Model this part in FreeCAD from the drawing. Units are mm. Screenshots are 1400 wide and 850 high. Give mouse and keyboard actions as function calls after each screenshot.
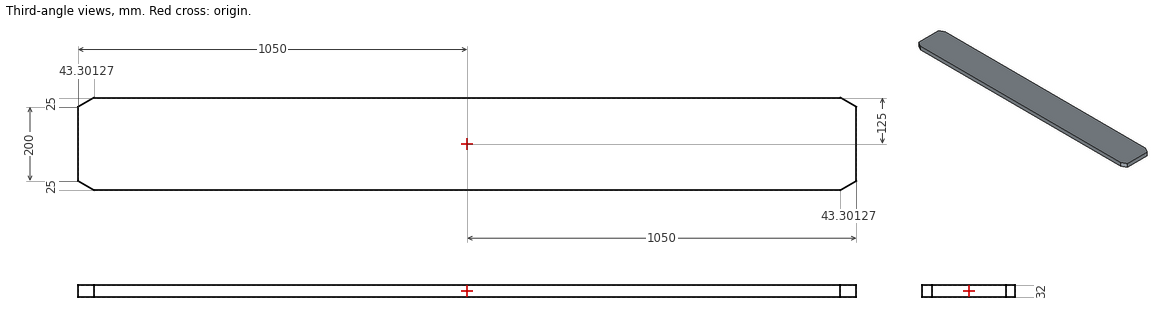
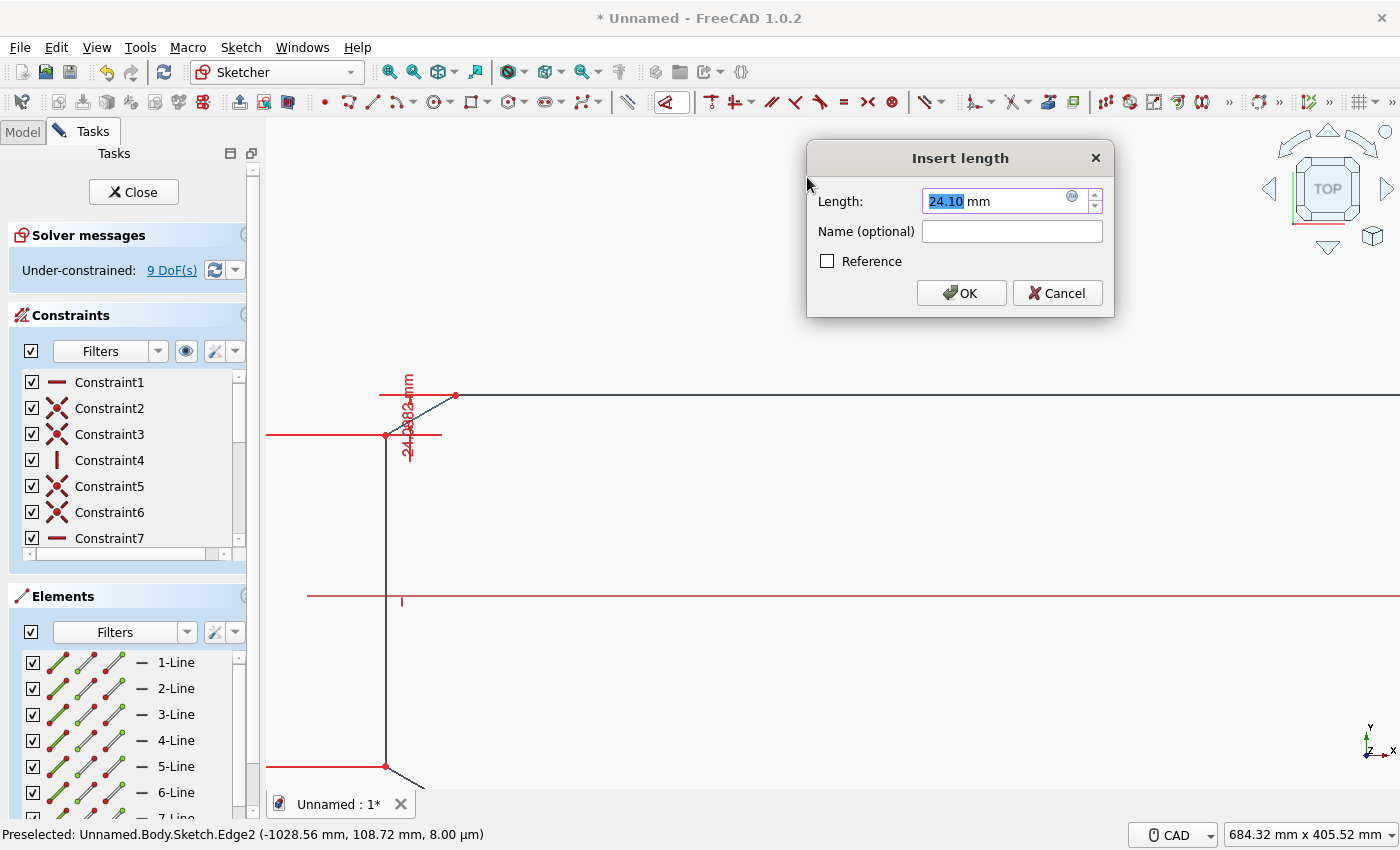
text(25)
key(Return)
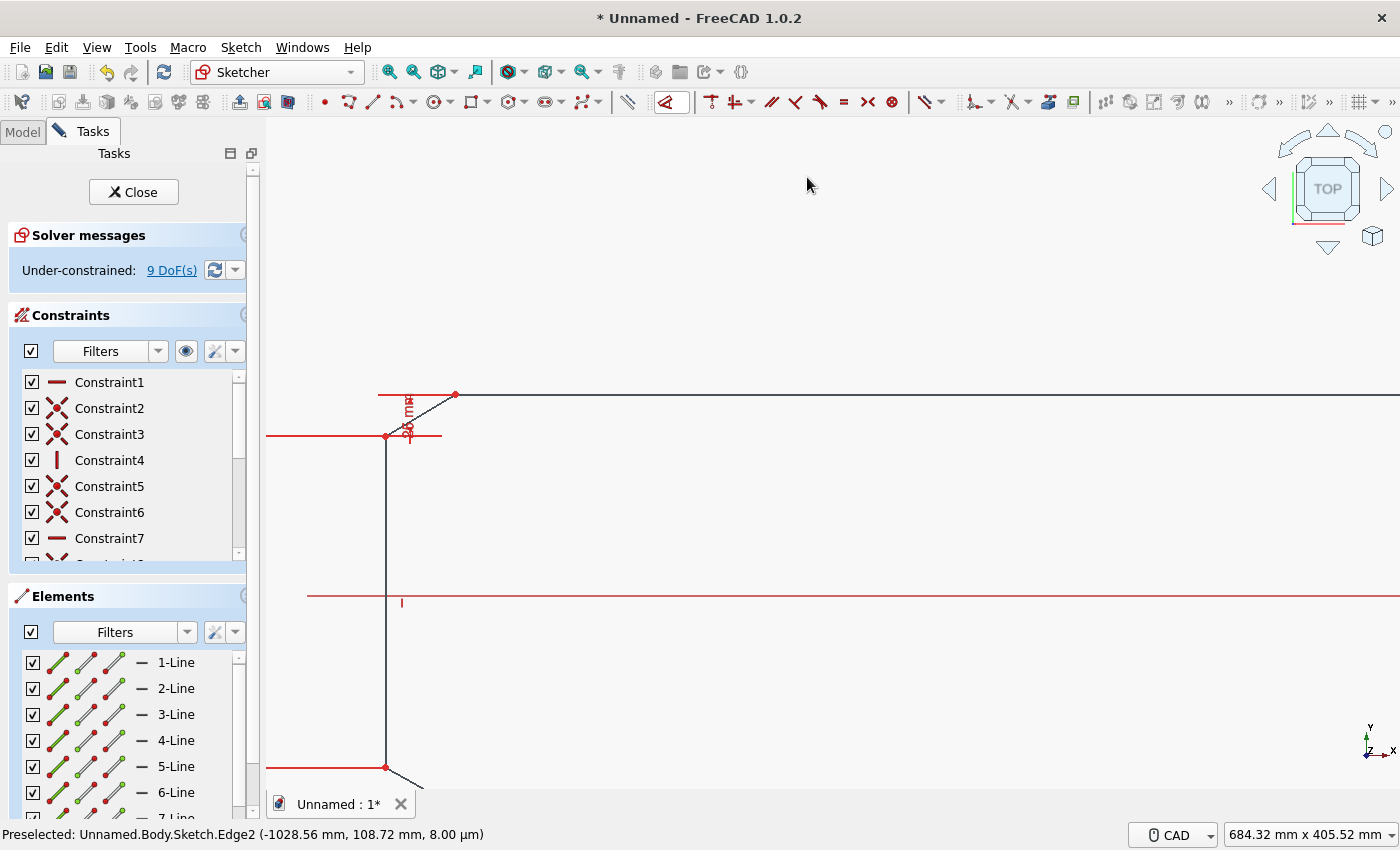
scroll(421, 417, down, 8)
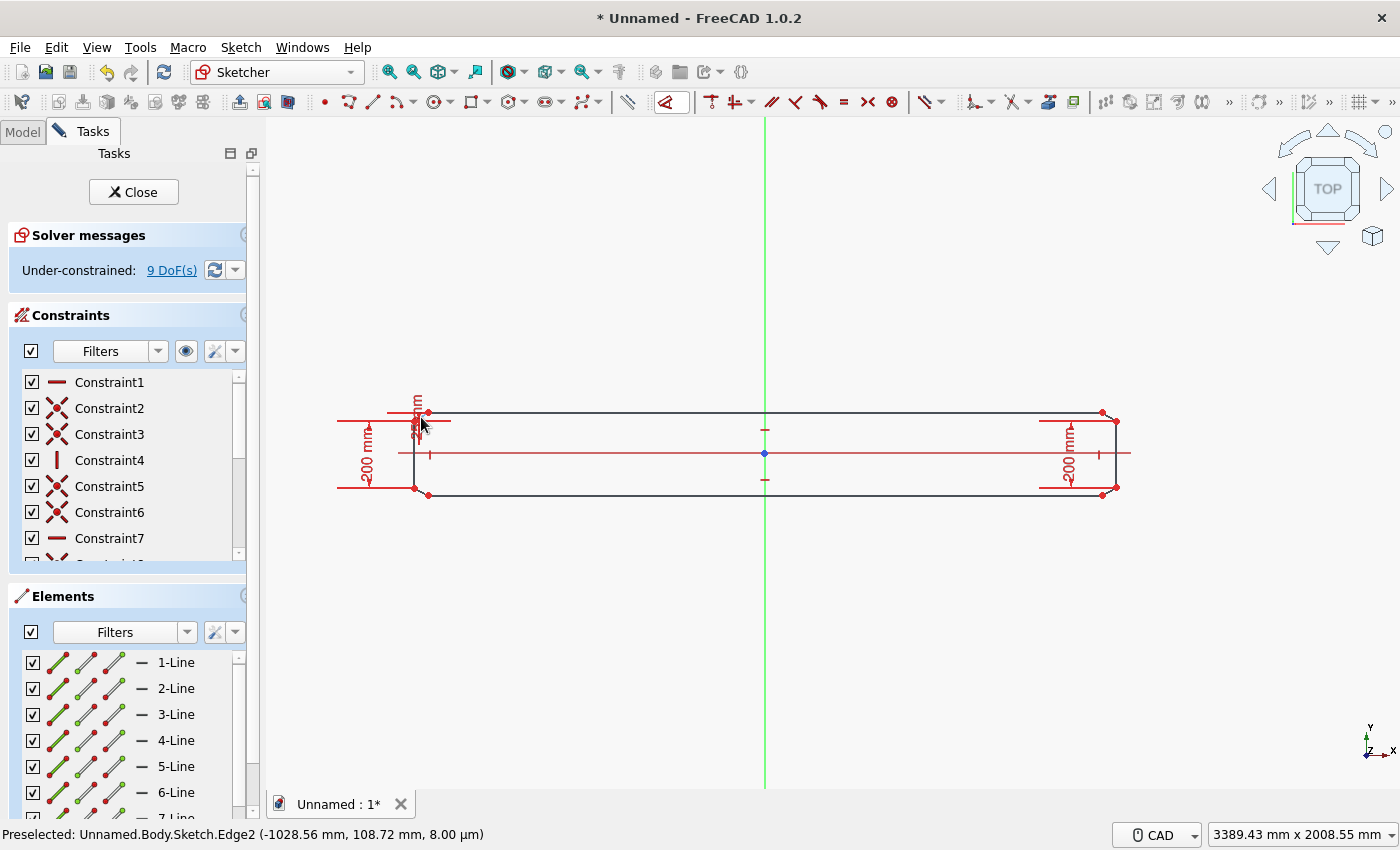
scroll(418, 491, up, 8)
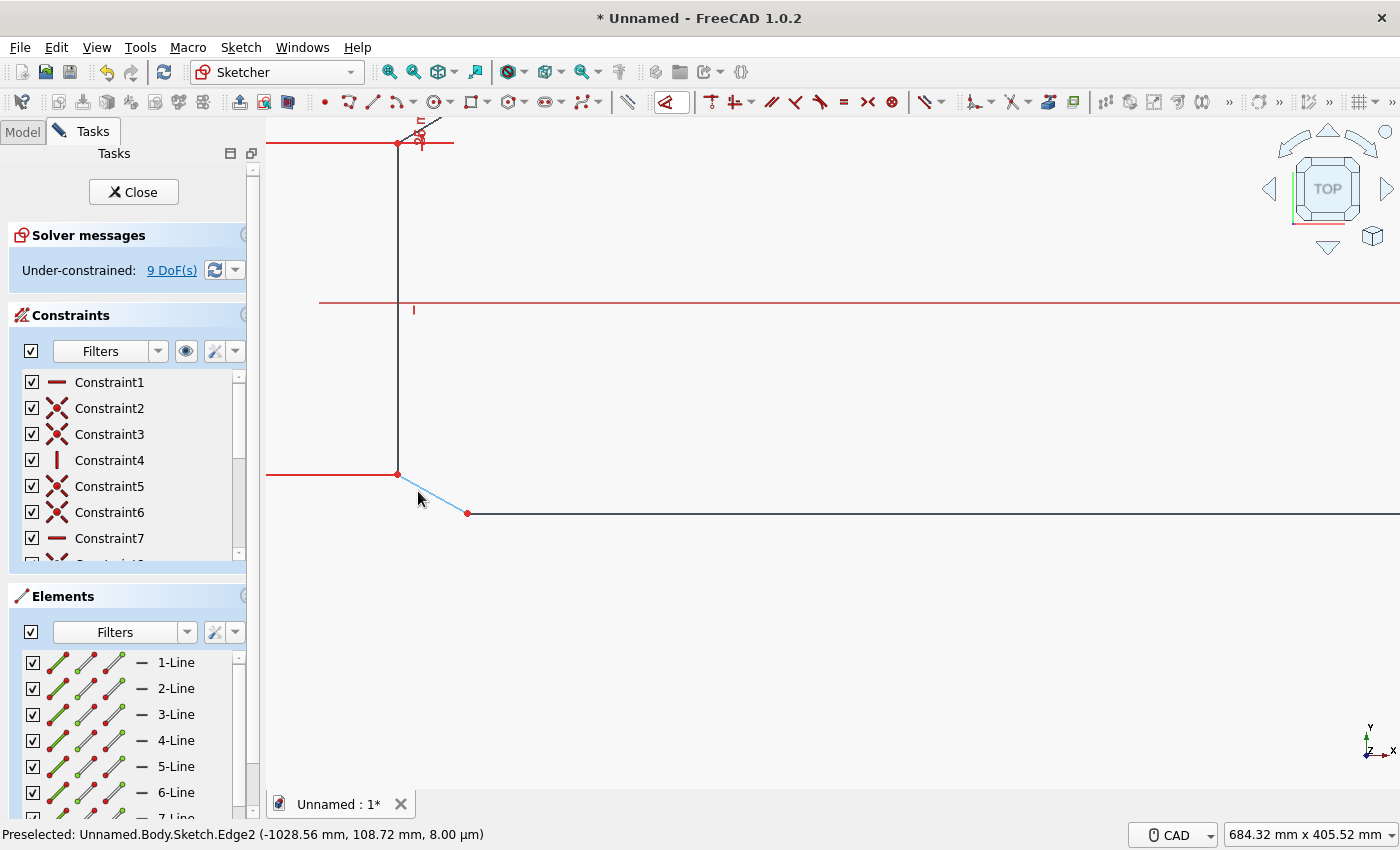
click(418, 486)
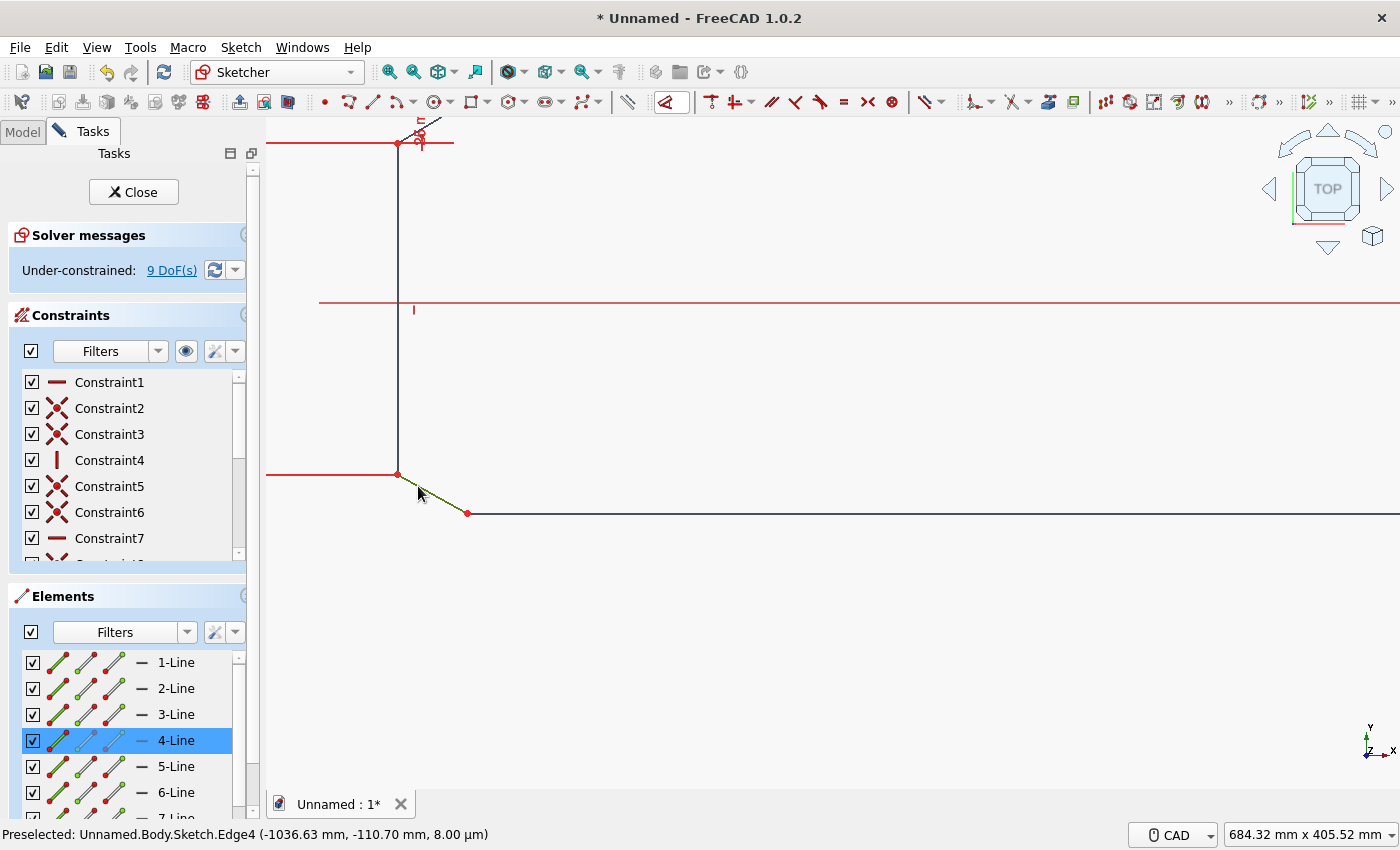
key(i)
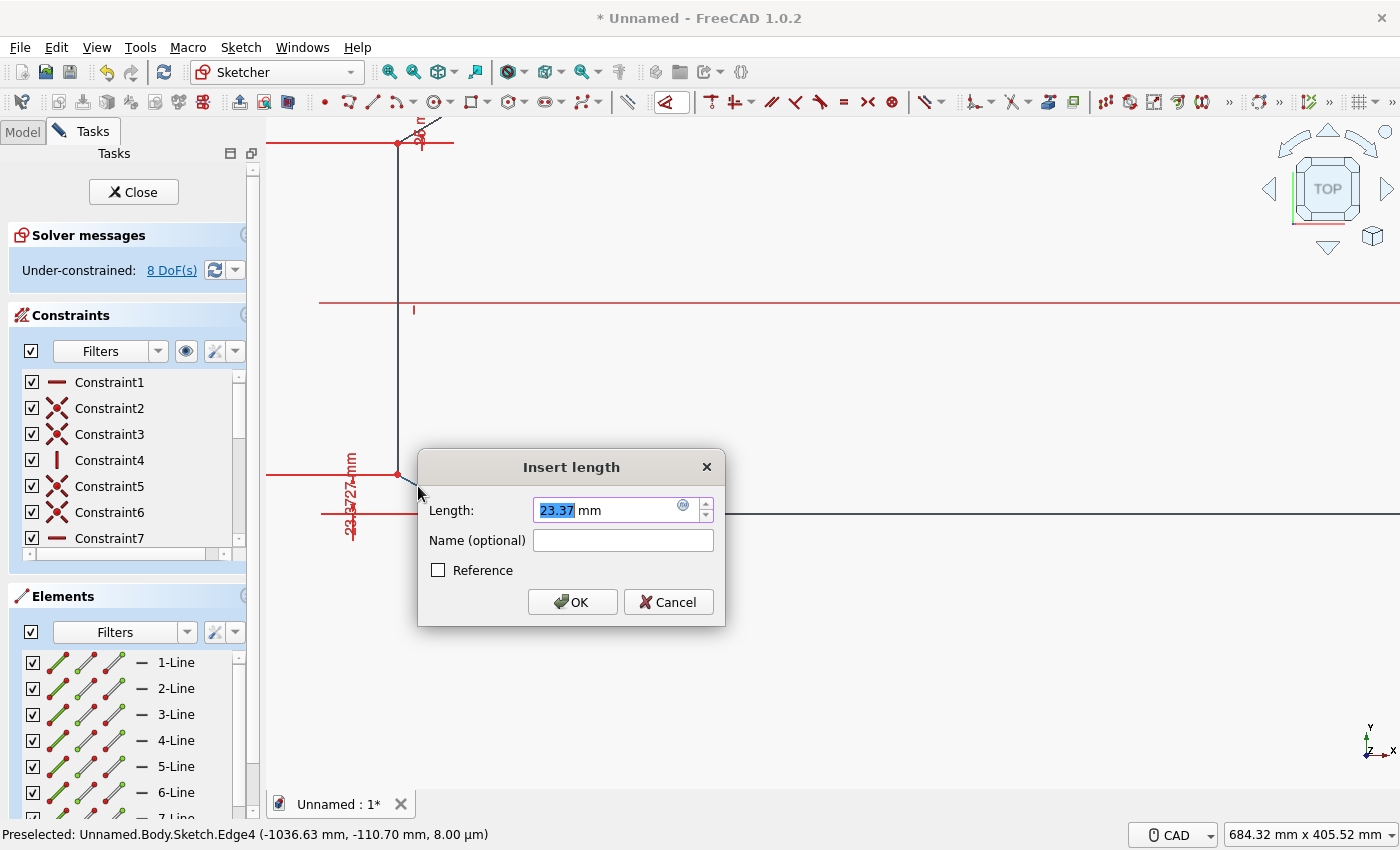
text(25)
key(Return)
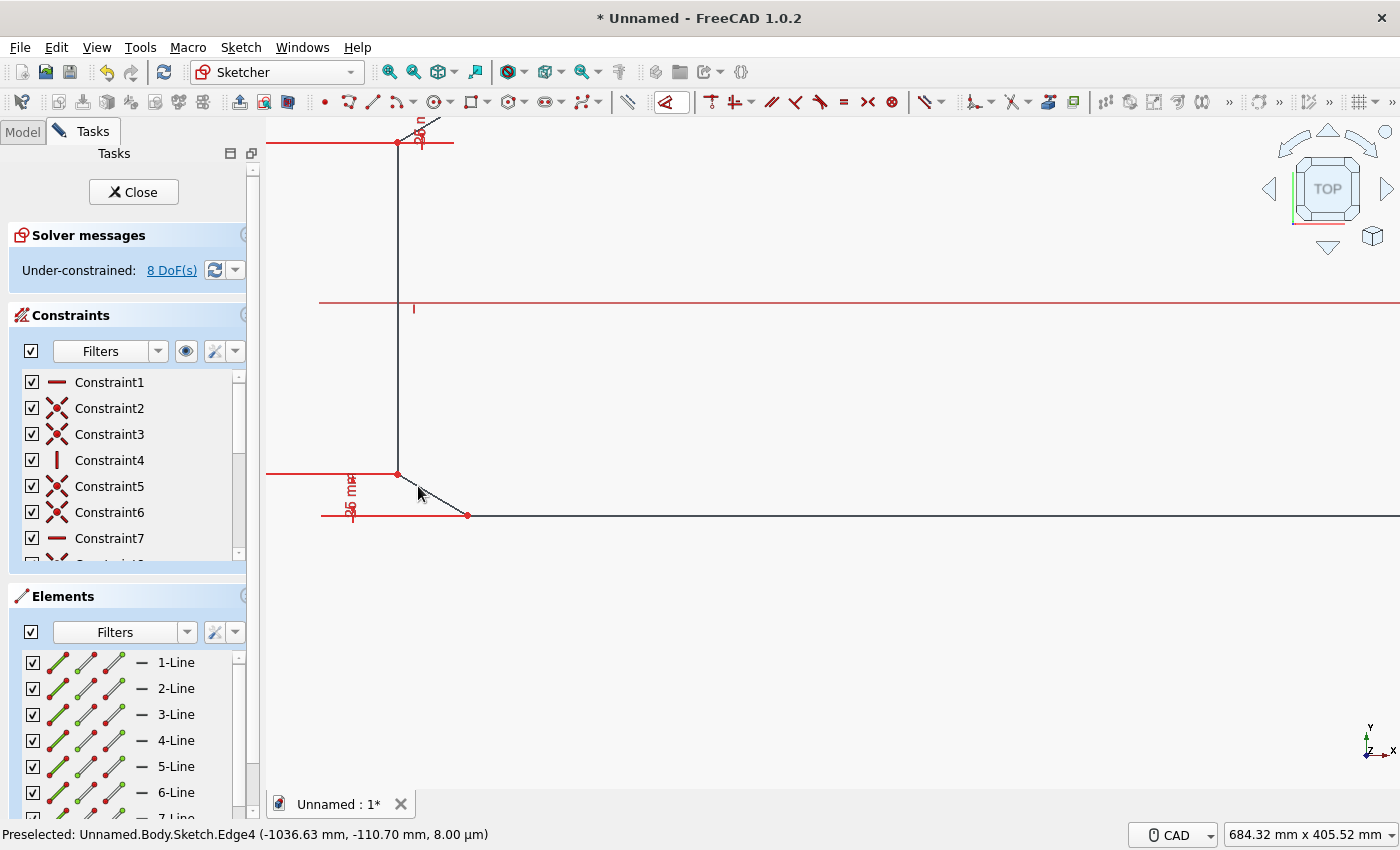
scroll(418, 491, down, 8)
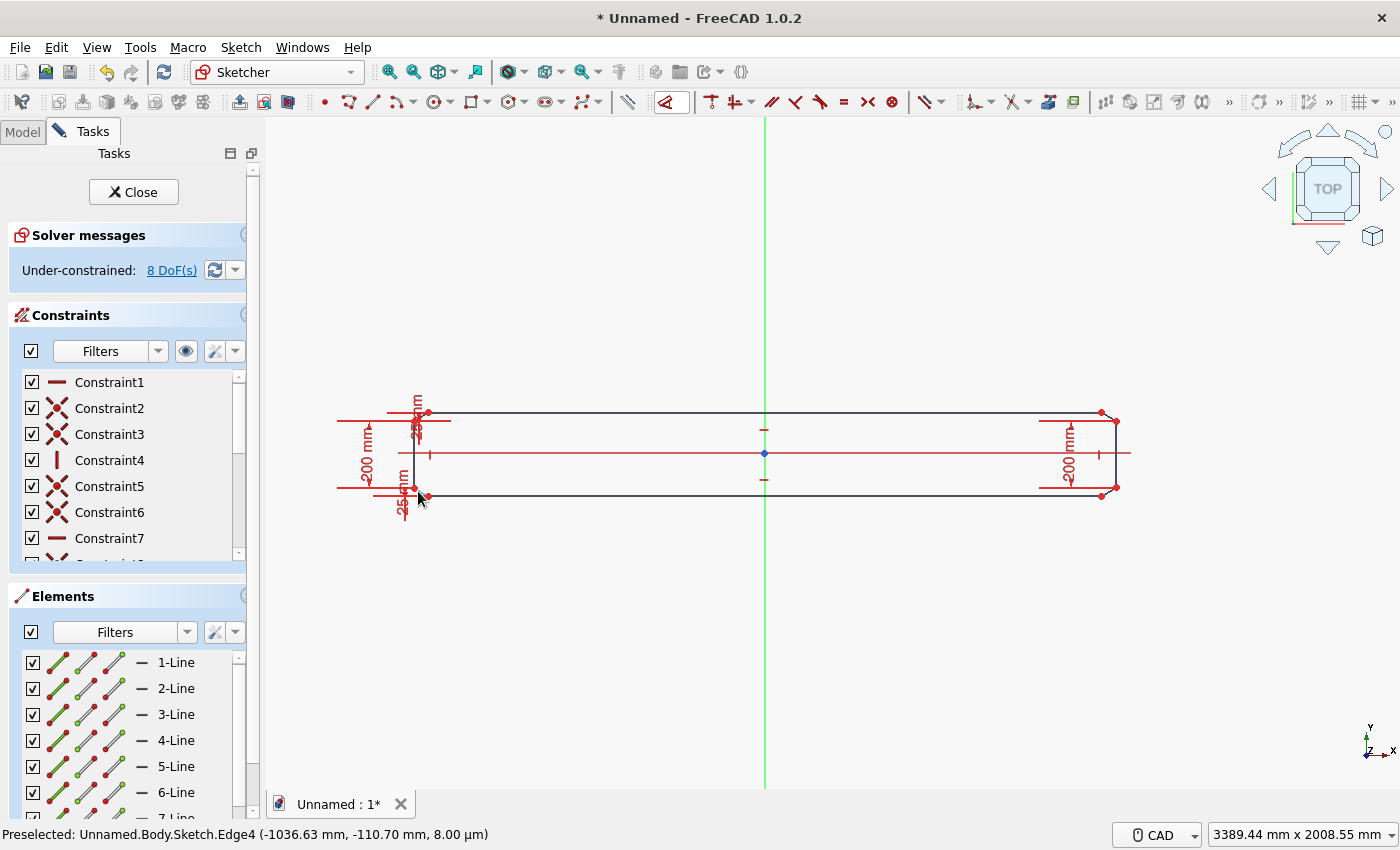
scroll(1106, 494, up, 8)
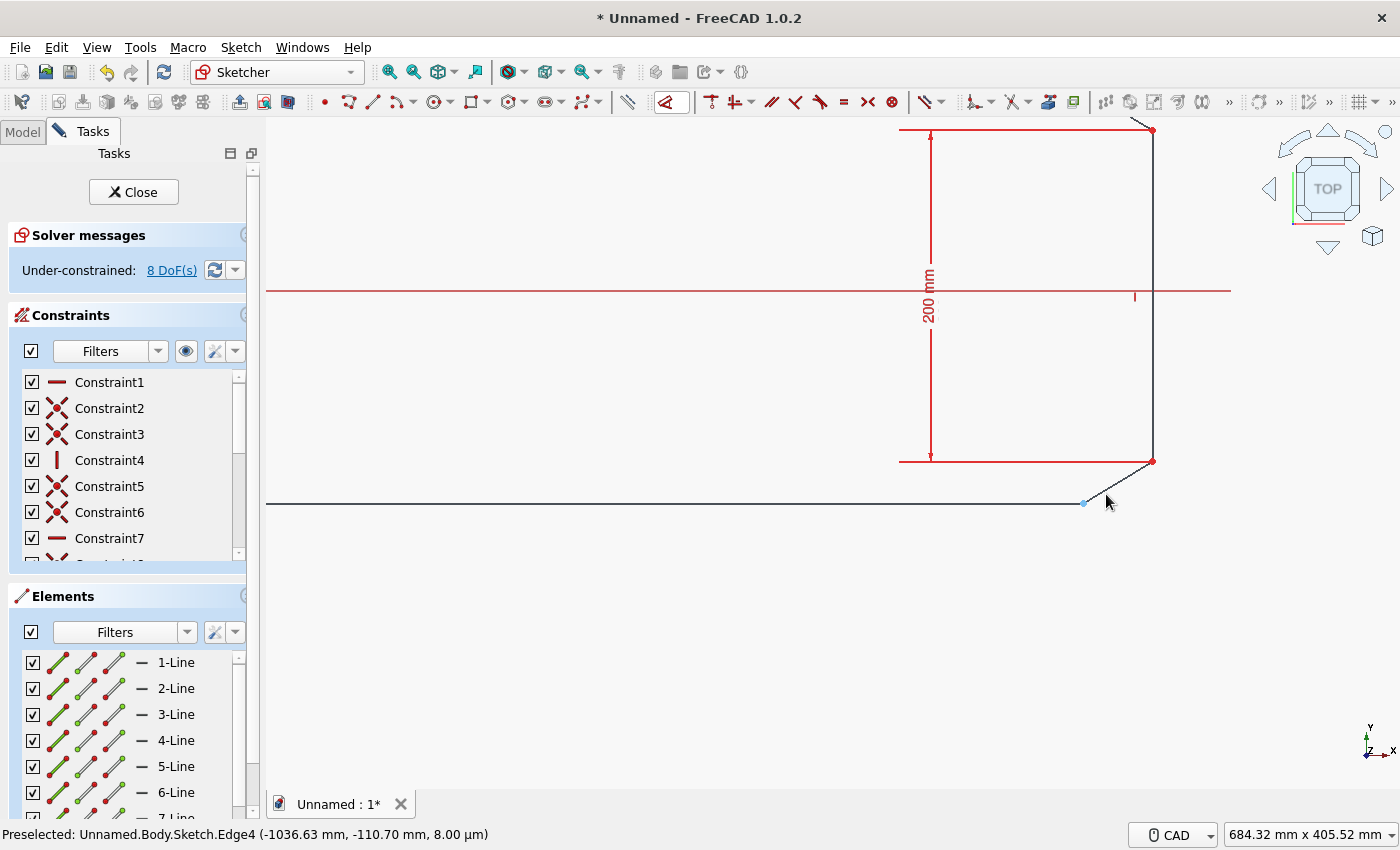
click(1104, 491)